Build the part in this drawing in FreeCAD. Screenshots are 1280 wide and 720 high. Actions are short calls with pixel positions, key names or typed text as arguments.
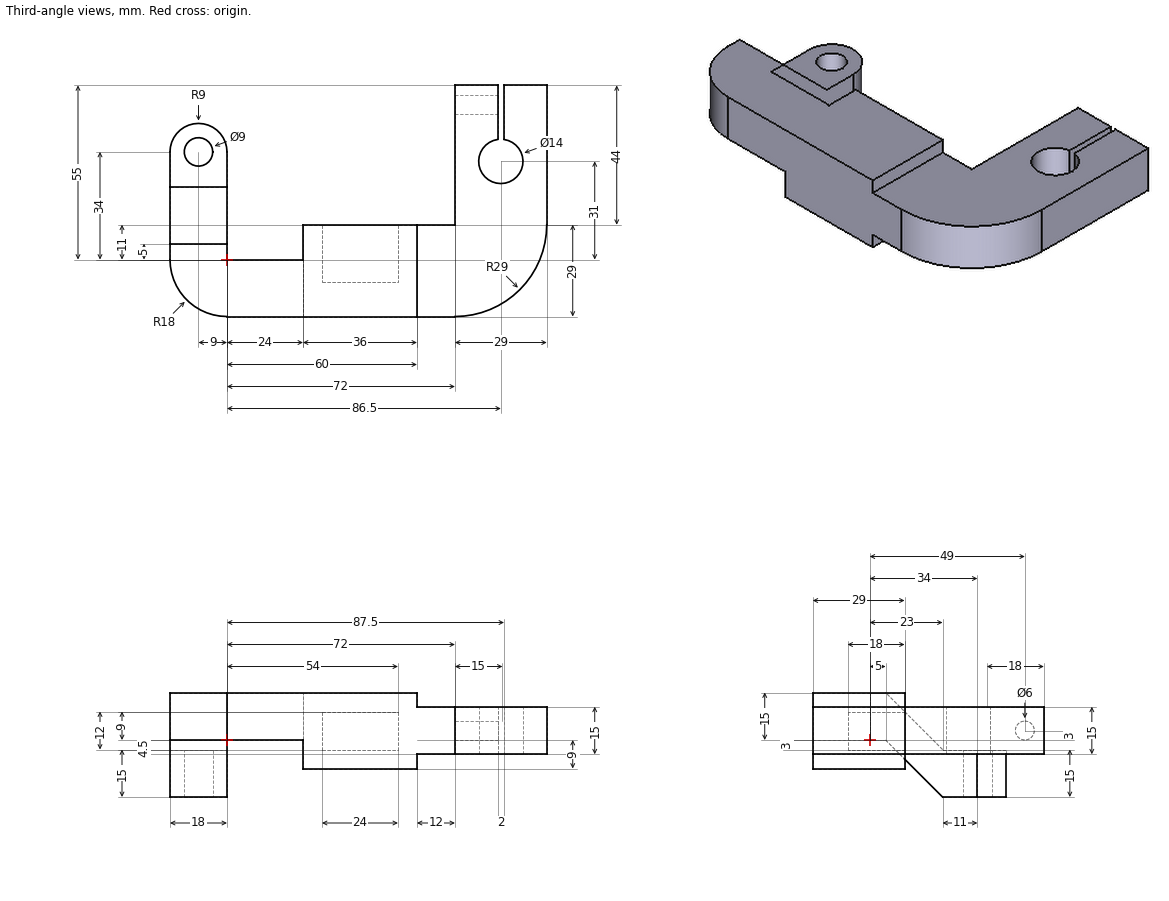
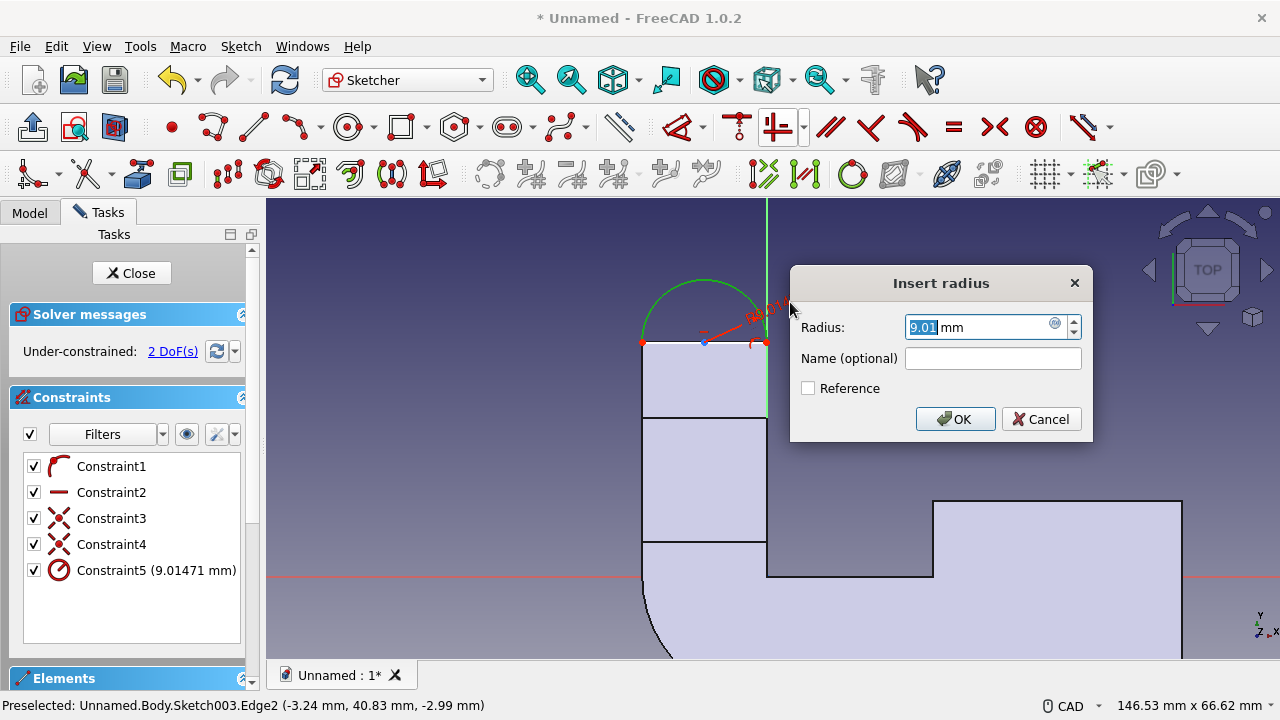
text(9)
key(Return)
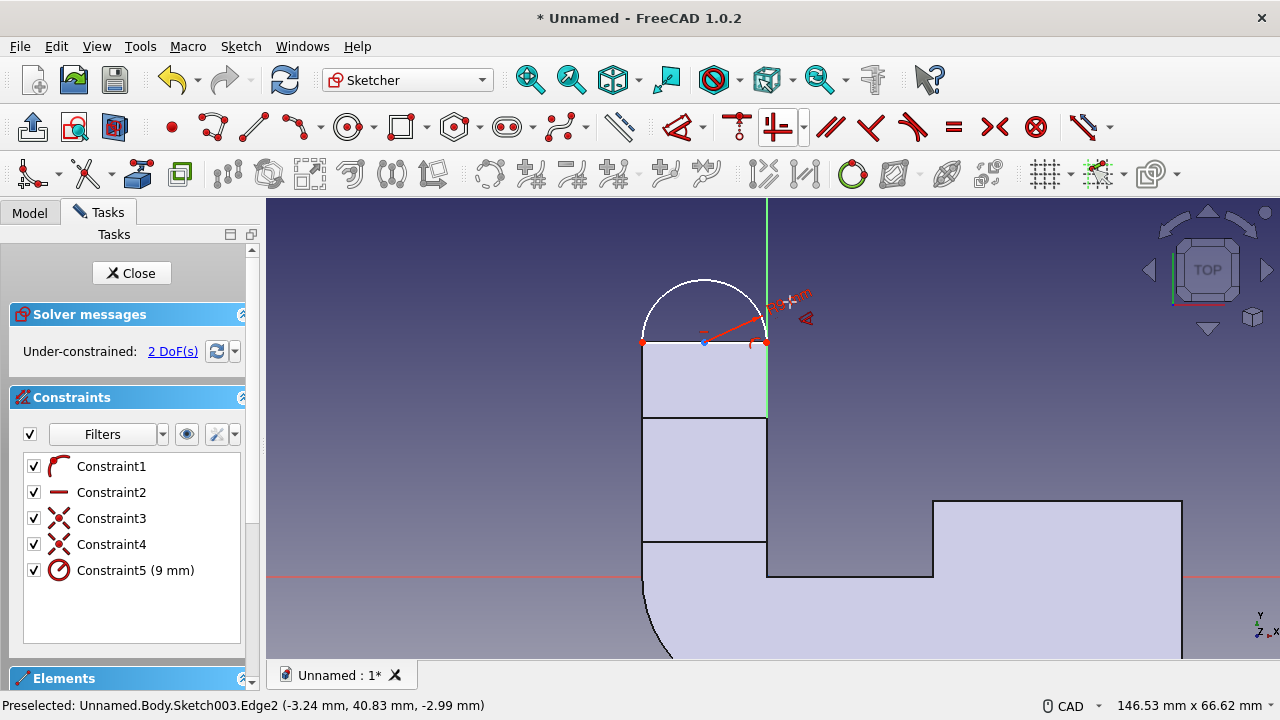
click(642, 343)
click(801, 460)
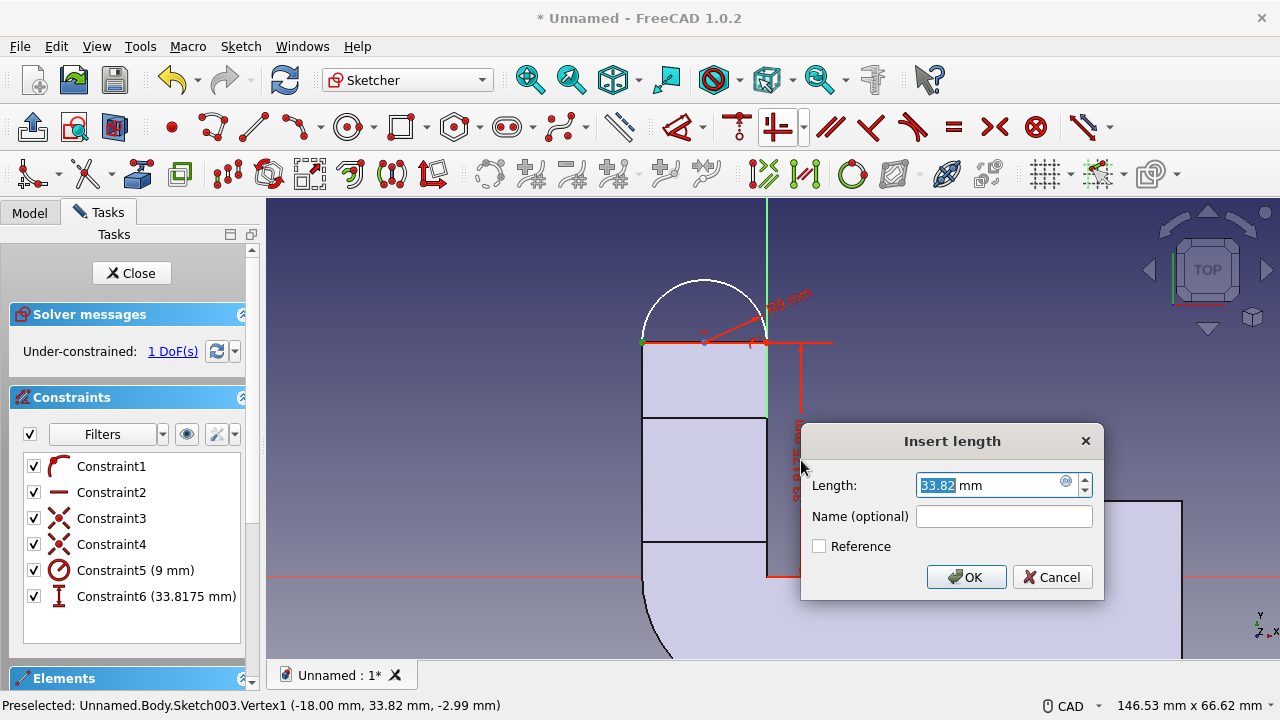
text(34)
key(Return)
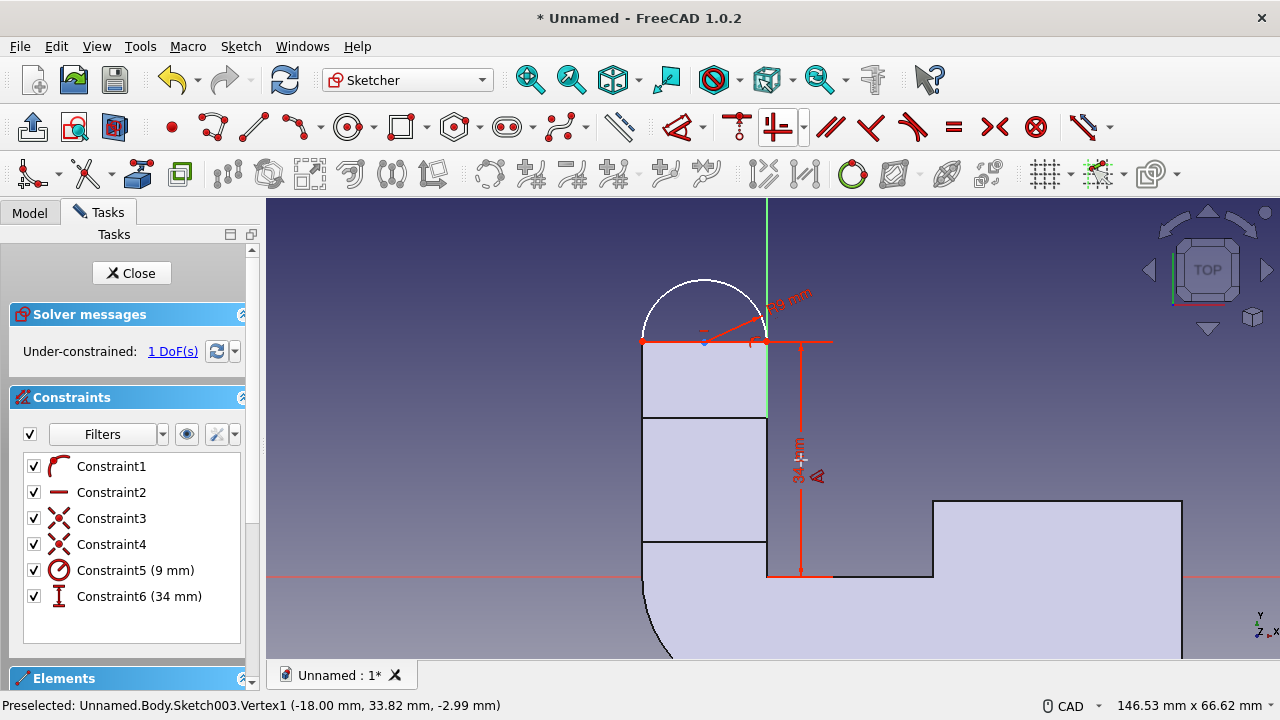
click(704, 342)
click(801, 406)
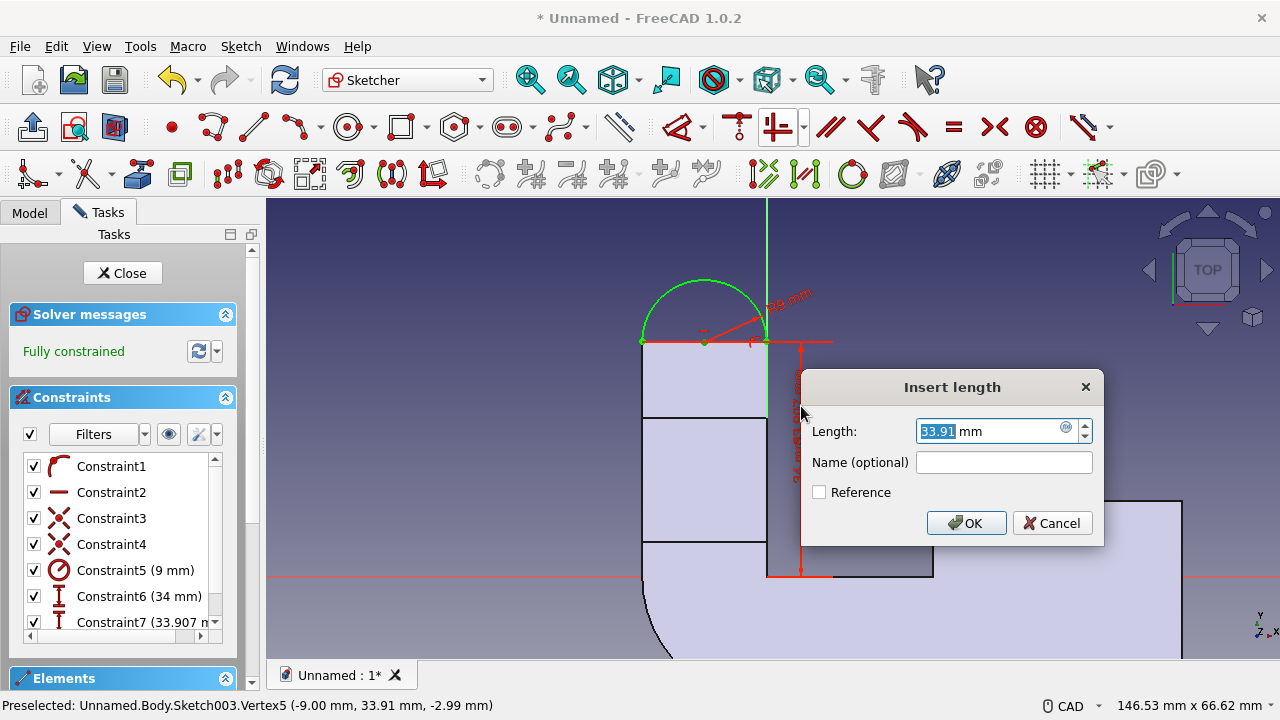
text(34)
key(Return)
key(Escape)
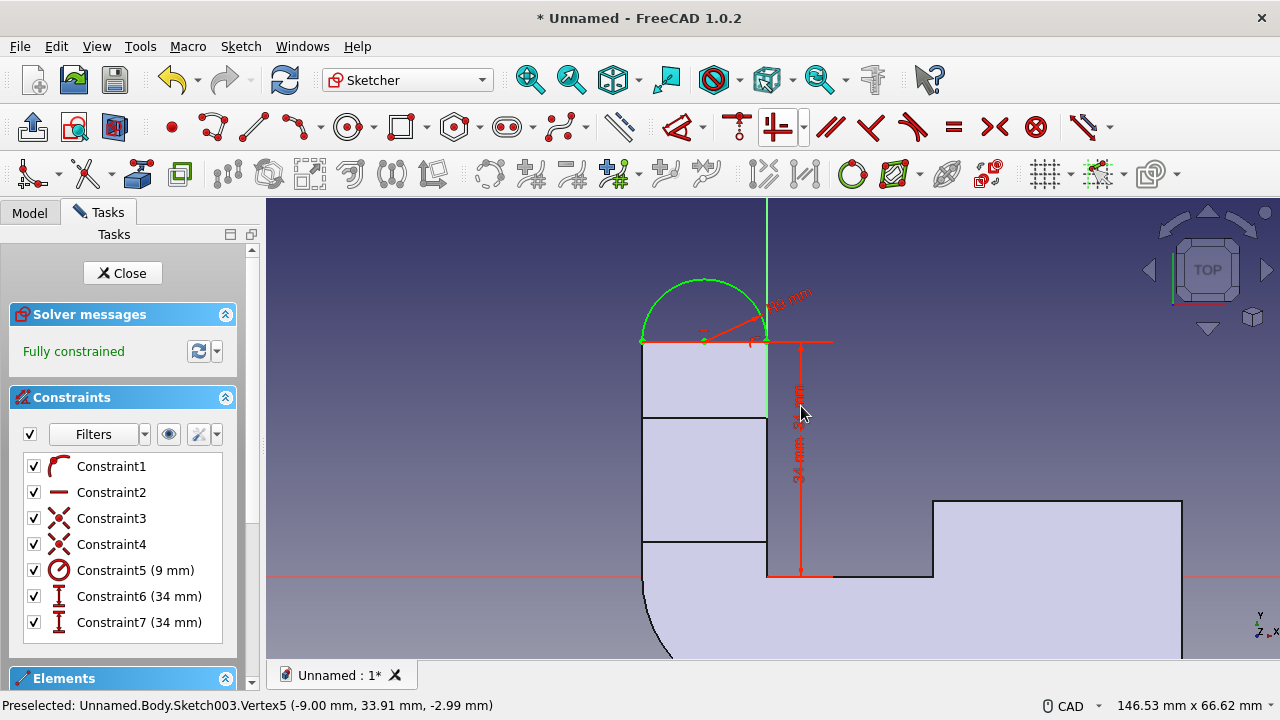
click(123, 273)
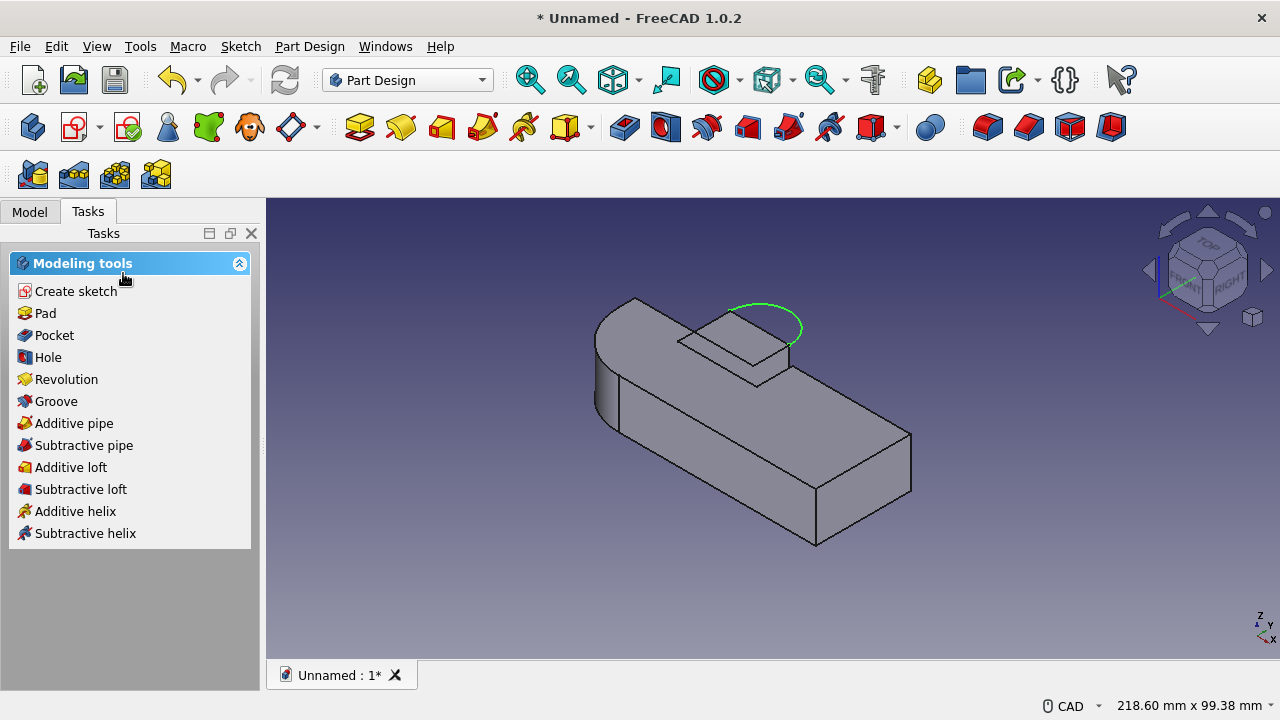
click(360, 128)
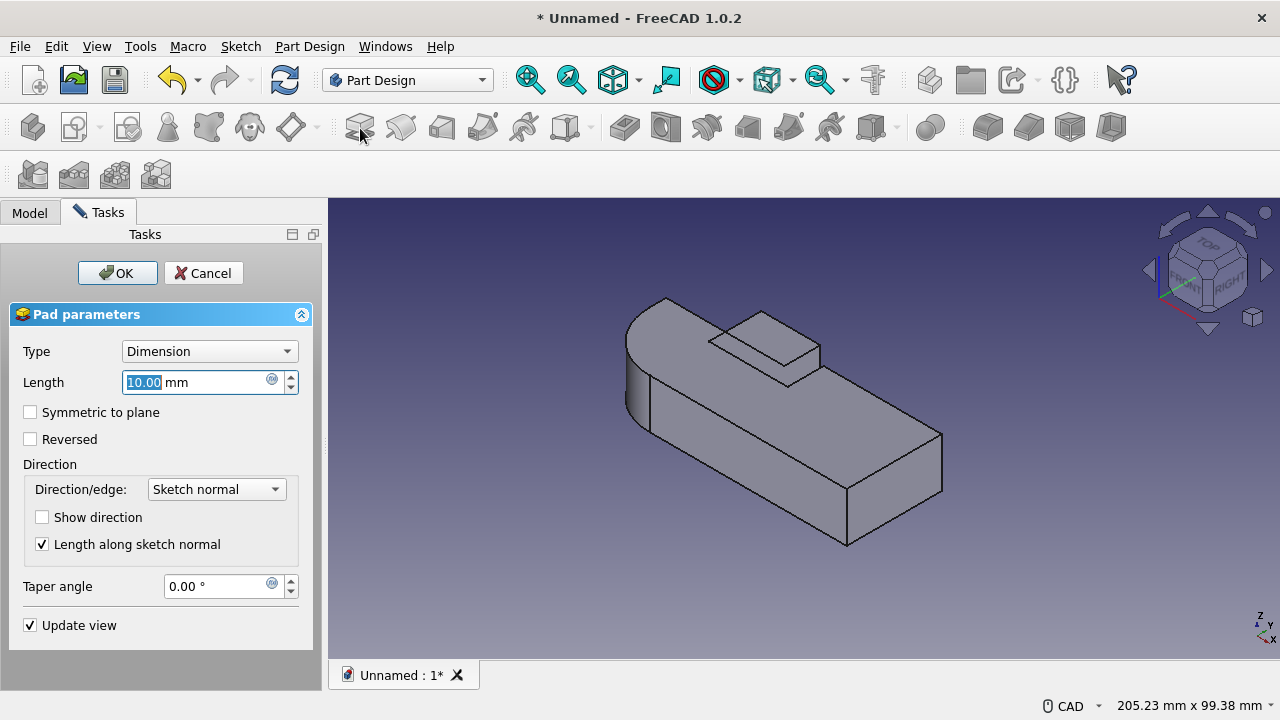
text(15)
key(Tab)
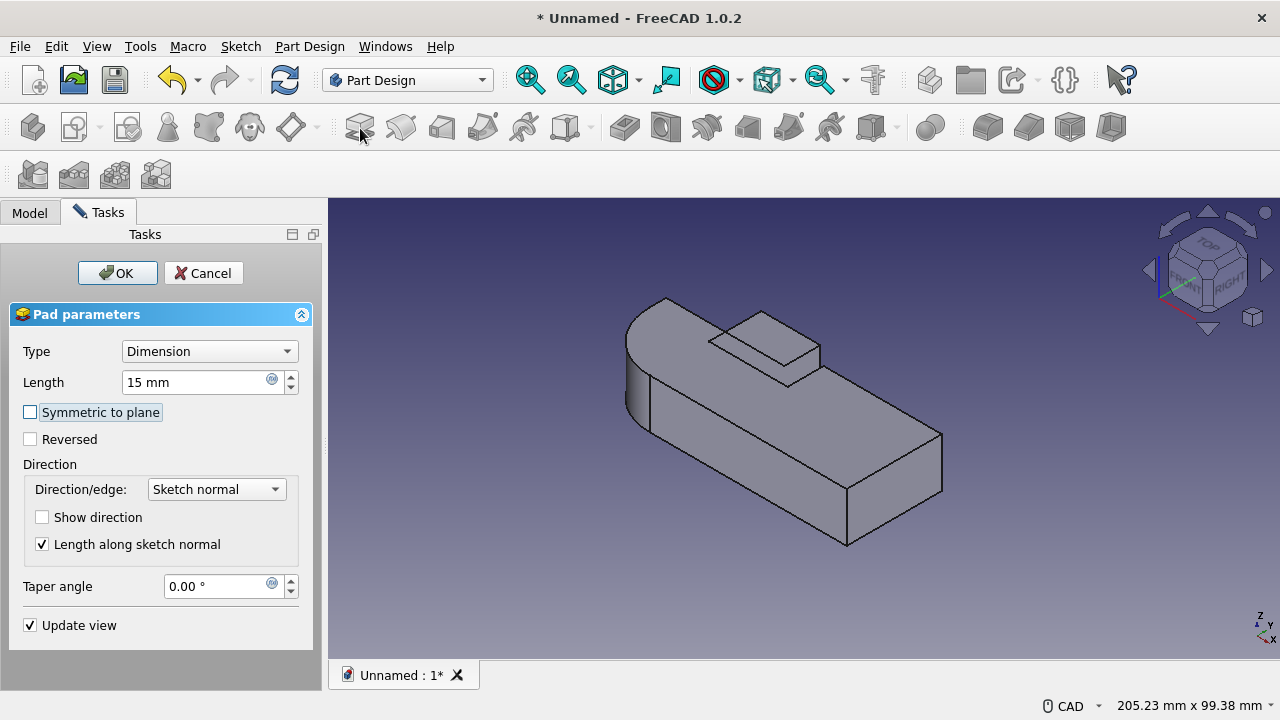
click(31, 439)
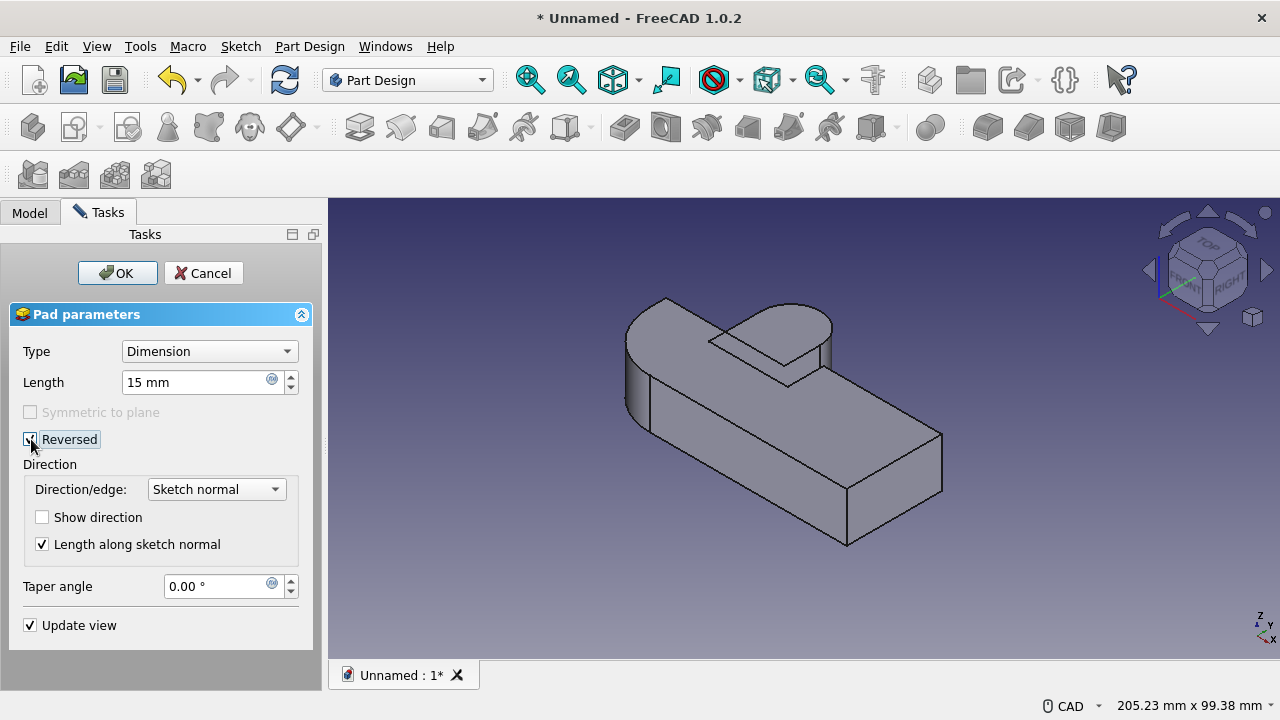
click(118, 273)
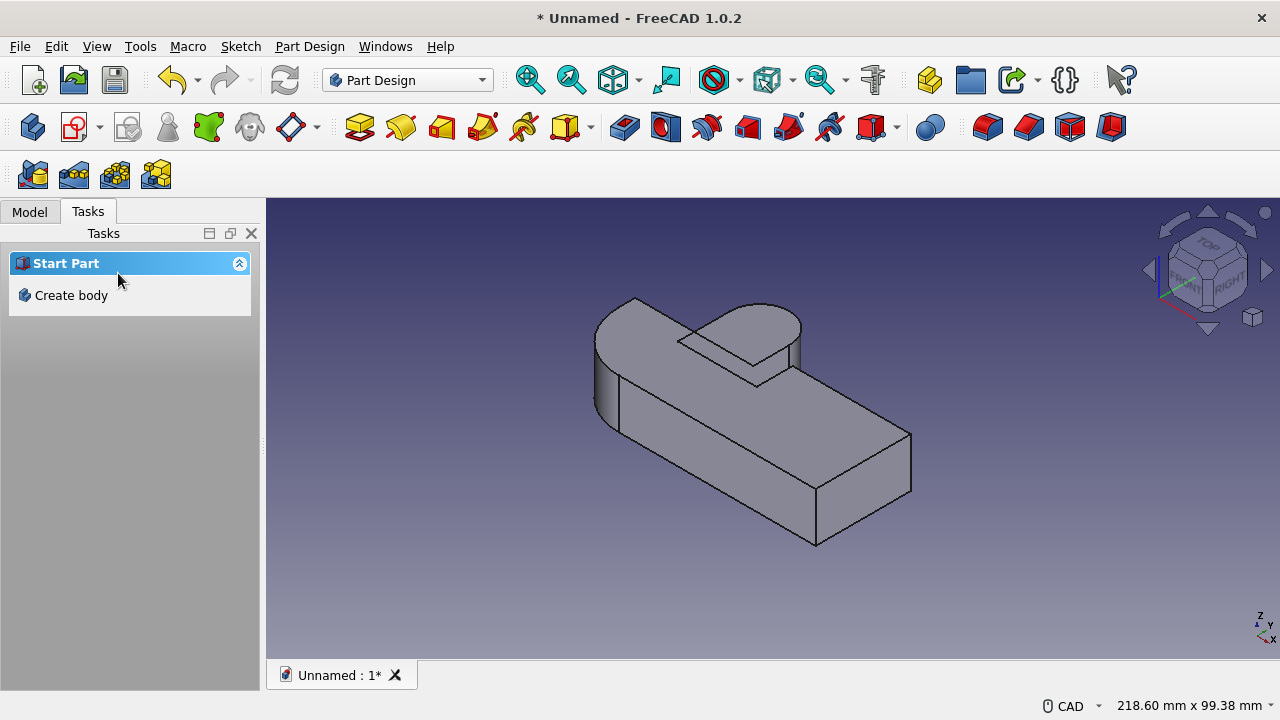
click(757, 329)